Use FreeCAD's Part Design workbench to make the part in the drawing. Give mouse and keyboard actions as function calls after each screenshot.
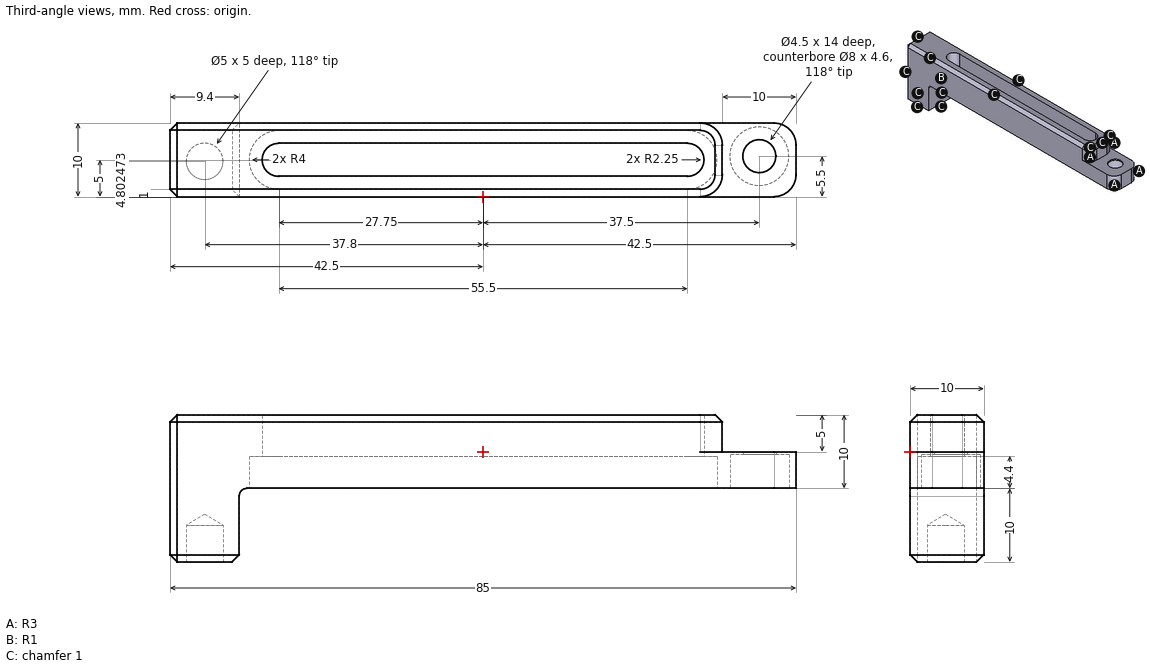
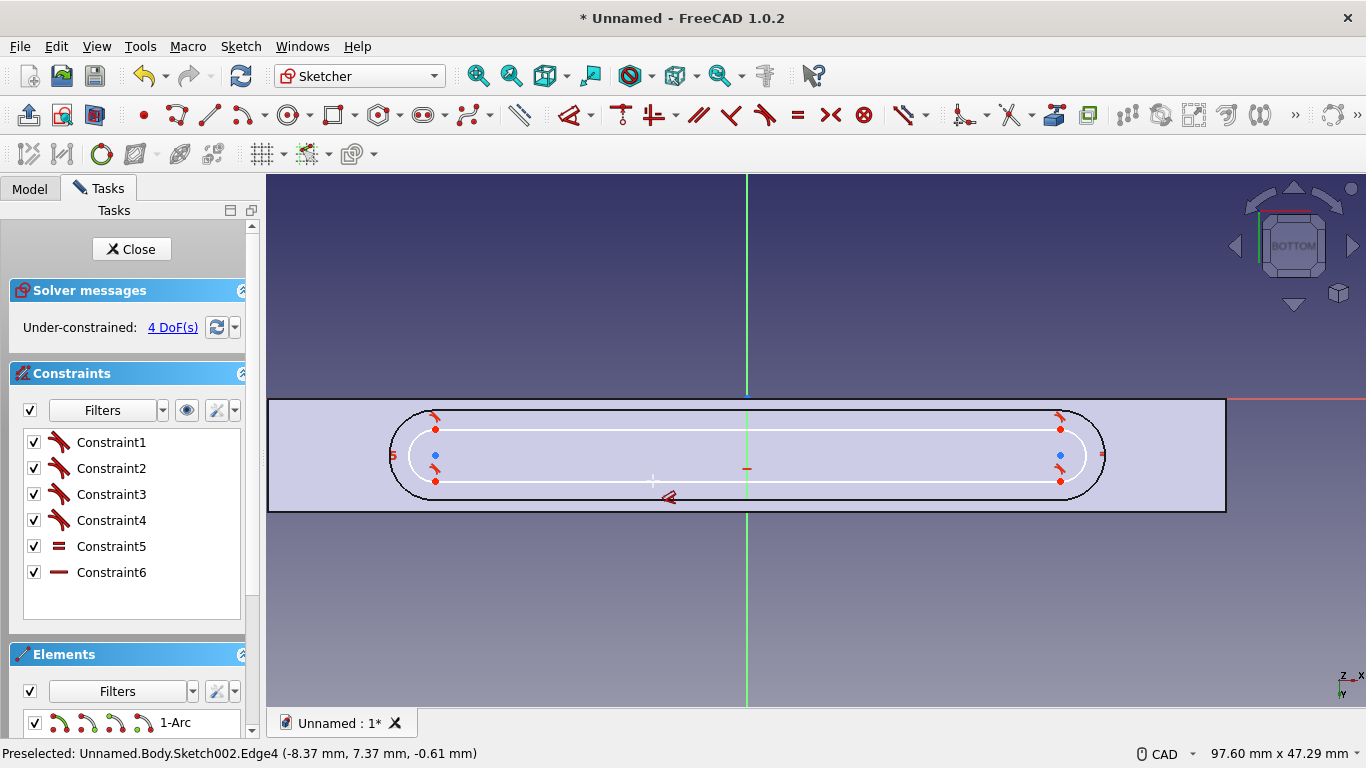
scroll(414, 441, up, 3)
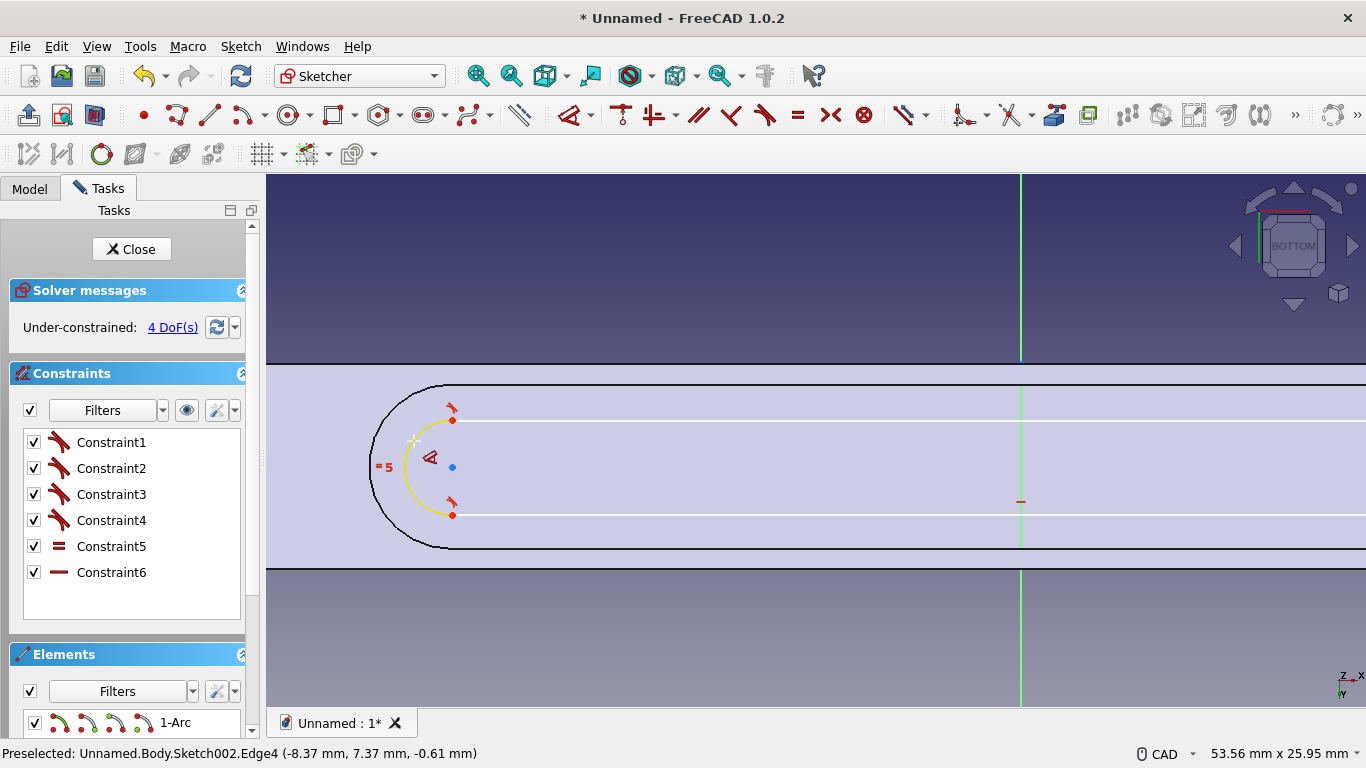
click(414, 440)
click(388, 421)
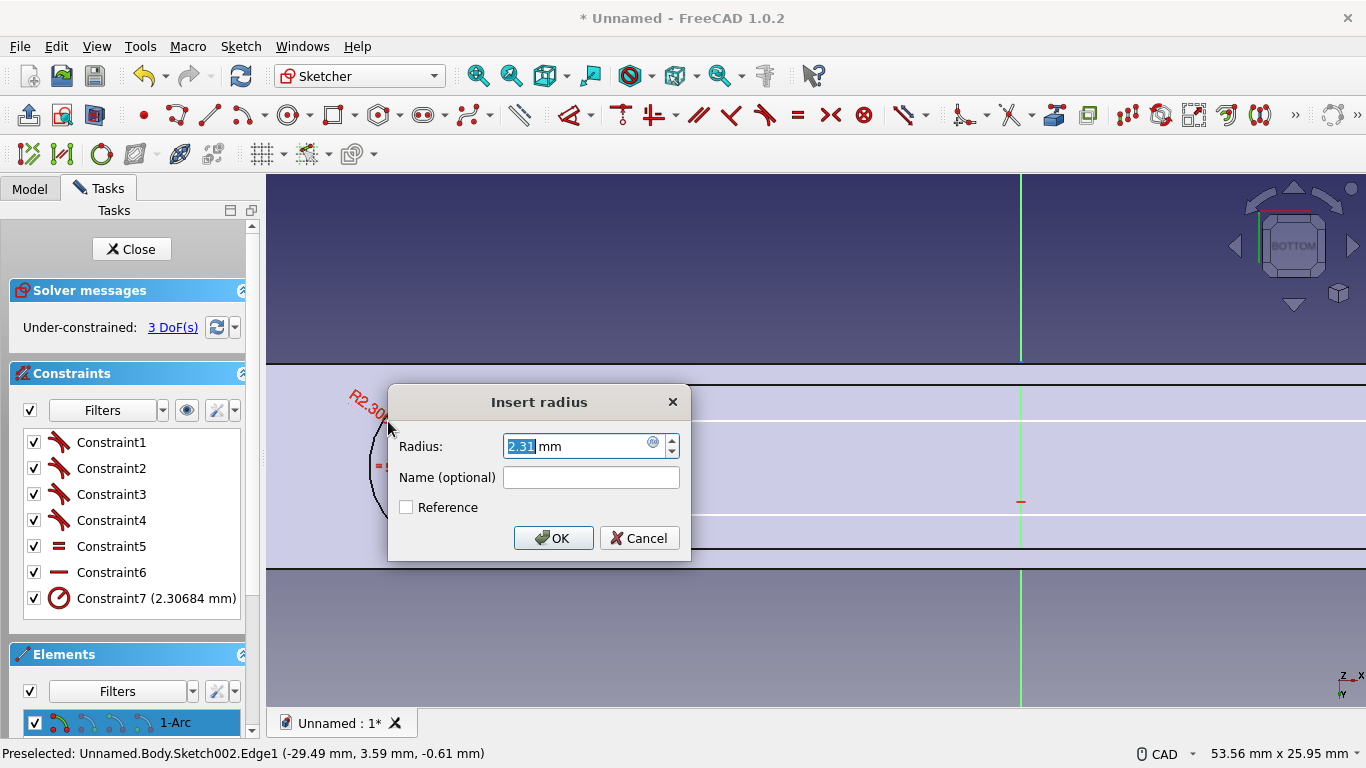
text(2.25)
key(Return)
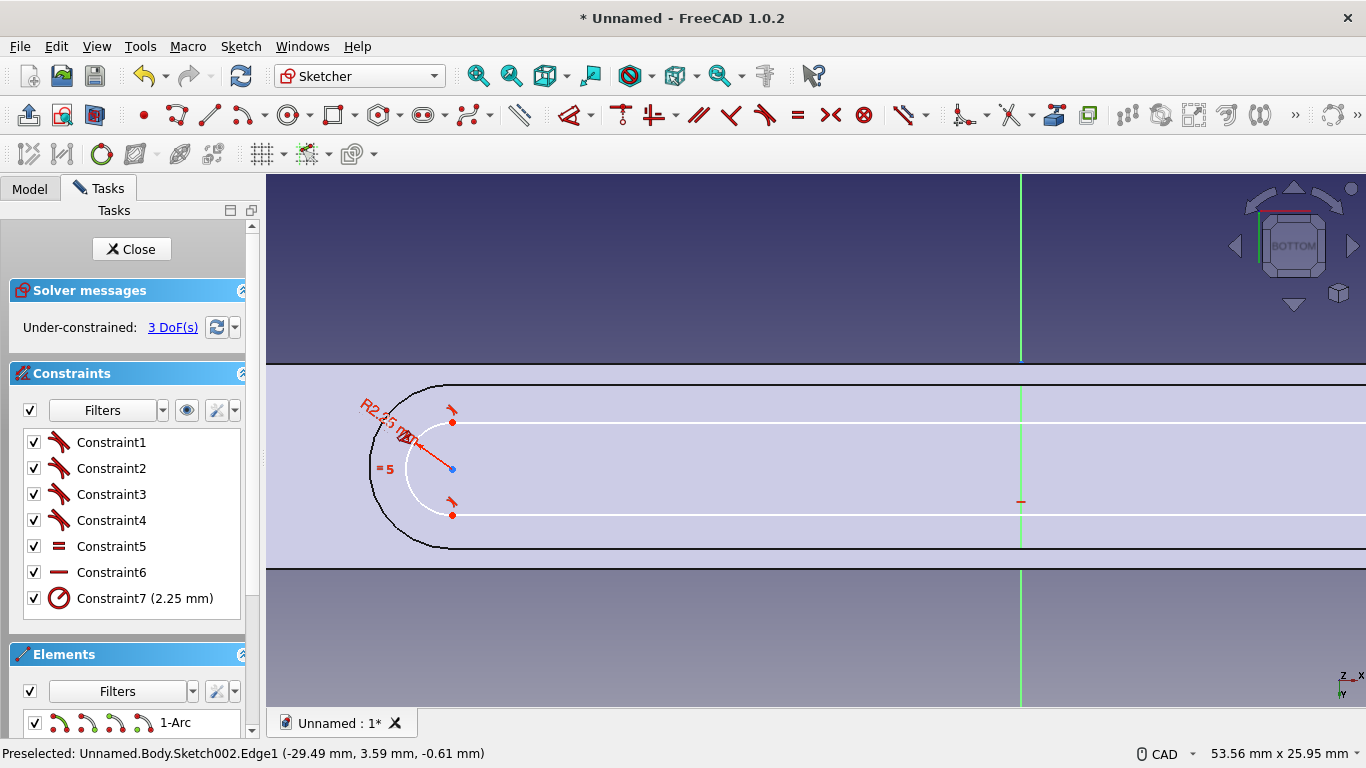
click(452, 469)
click(418, 392)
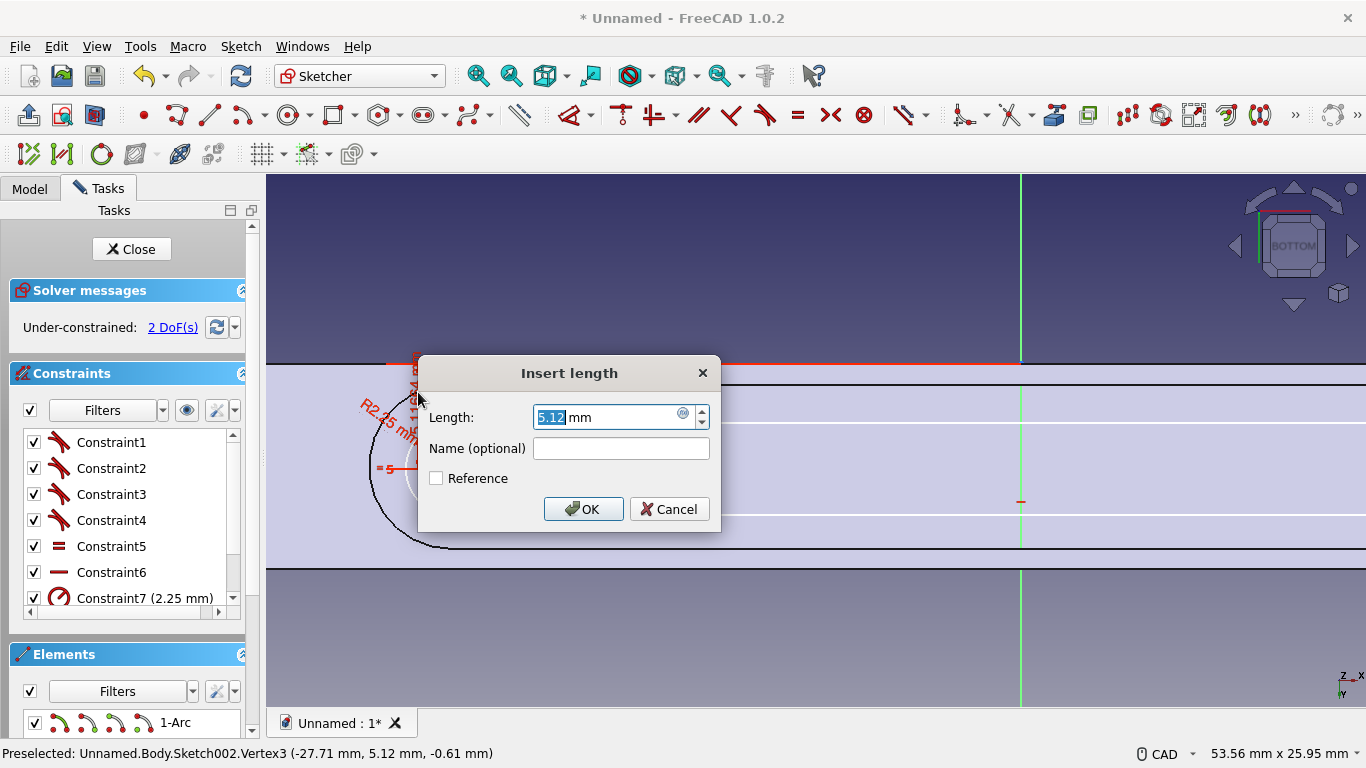
text(5)
key(Return)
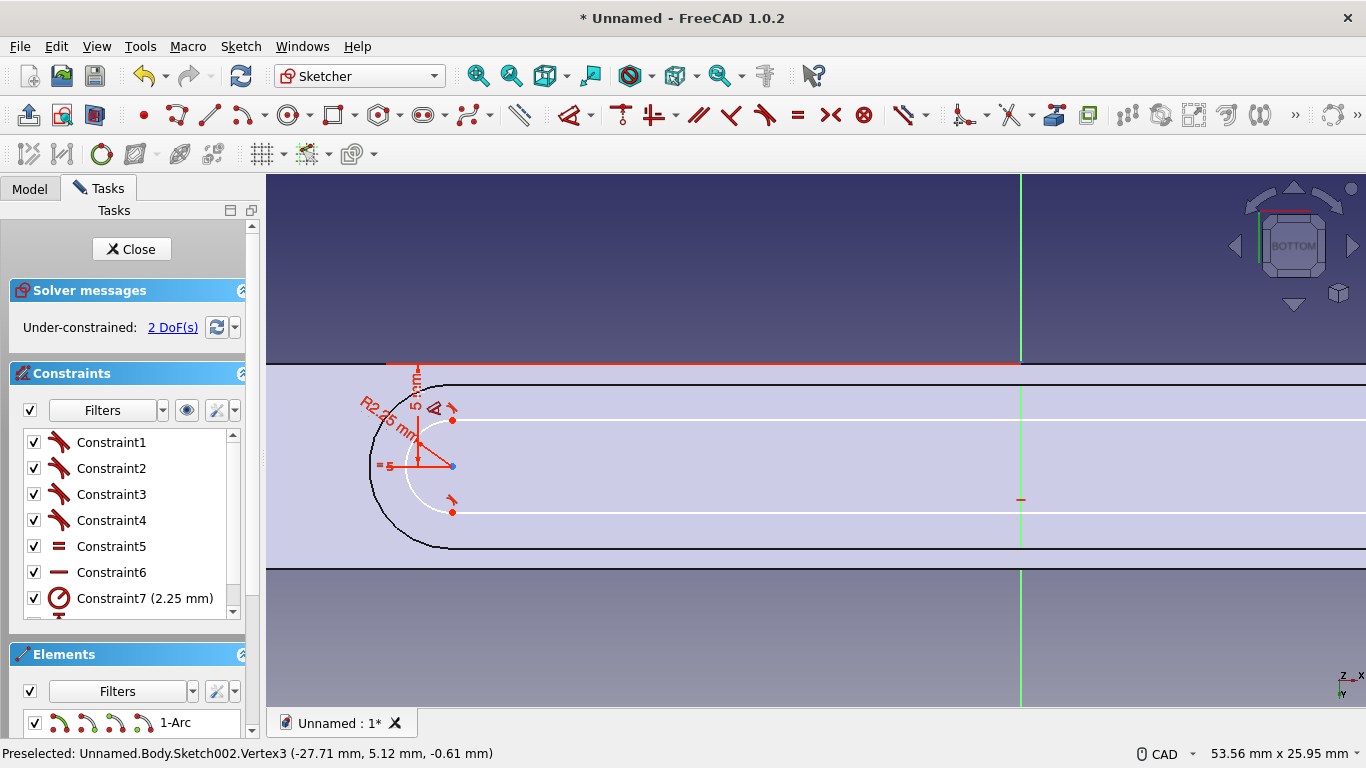
click(794, 420)
click(827, 386)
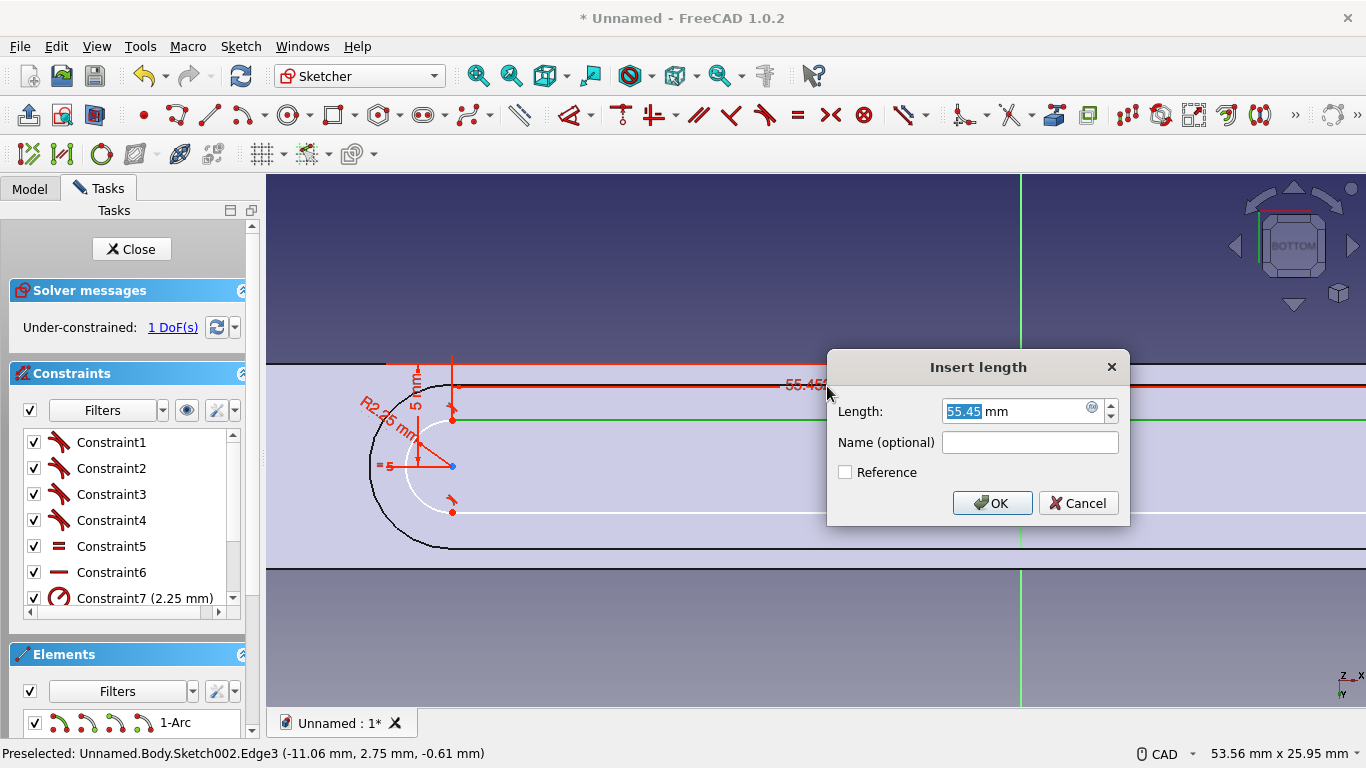
text(55.5)
key(Return)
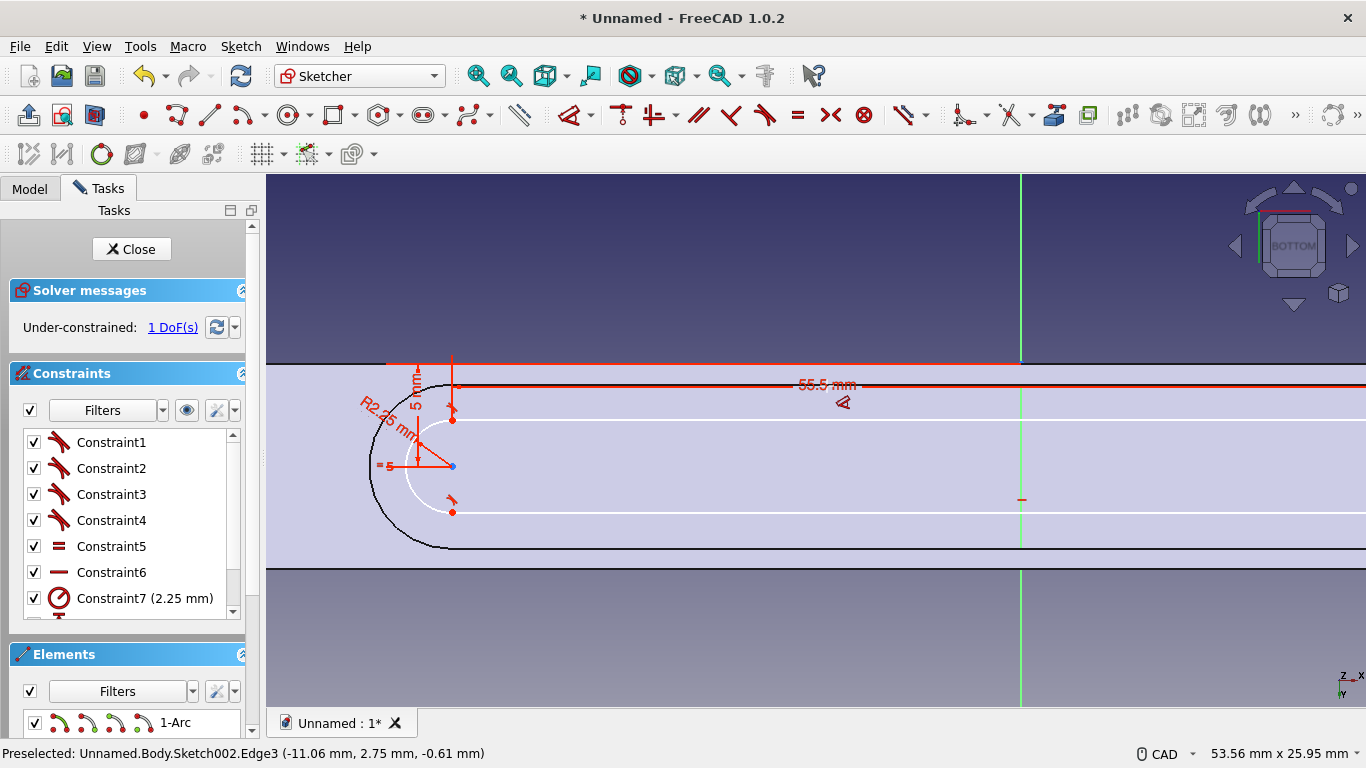
click(452, 420)
click(737, 330)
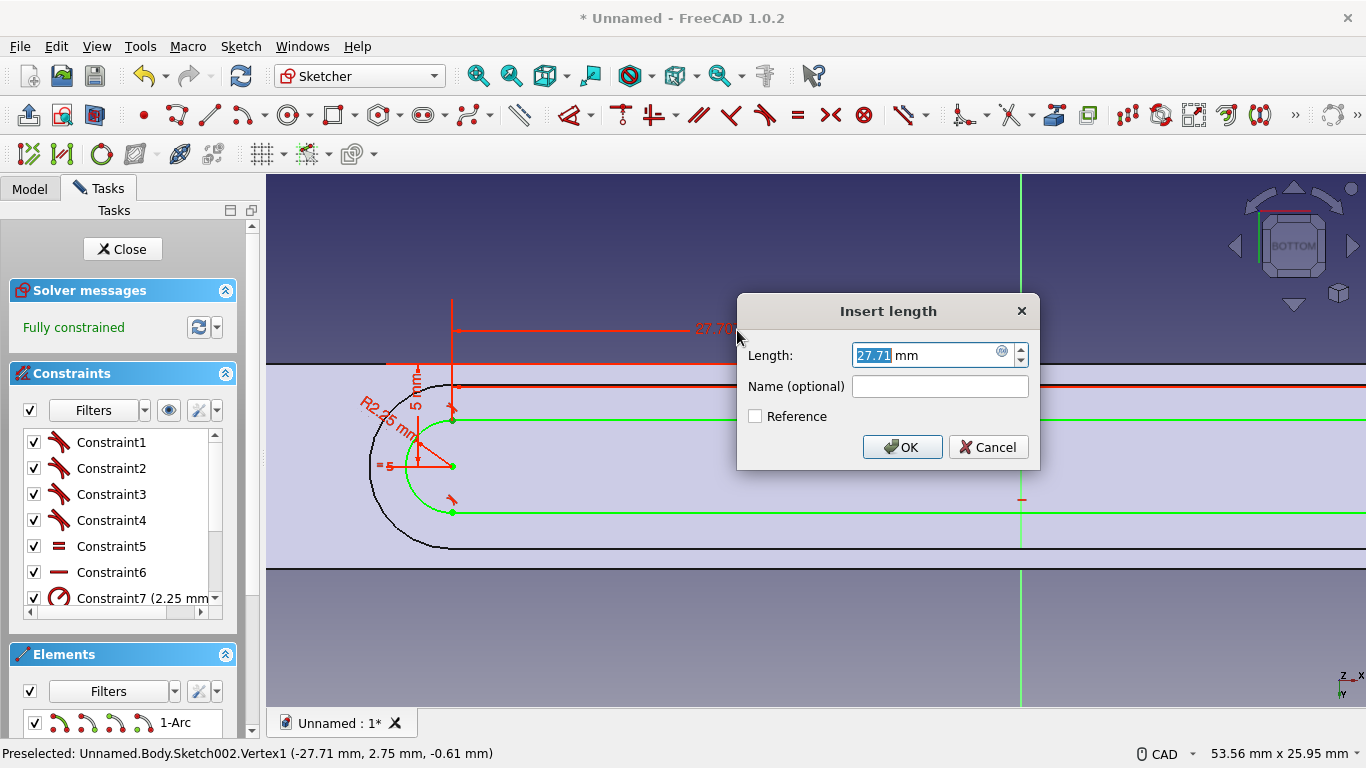
text(27.75)
key(Return)
key(Escape)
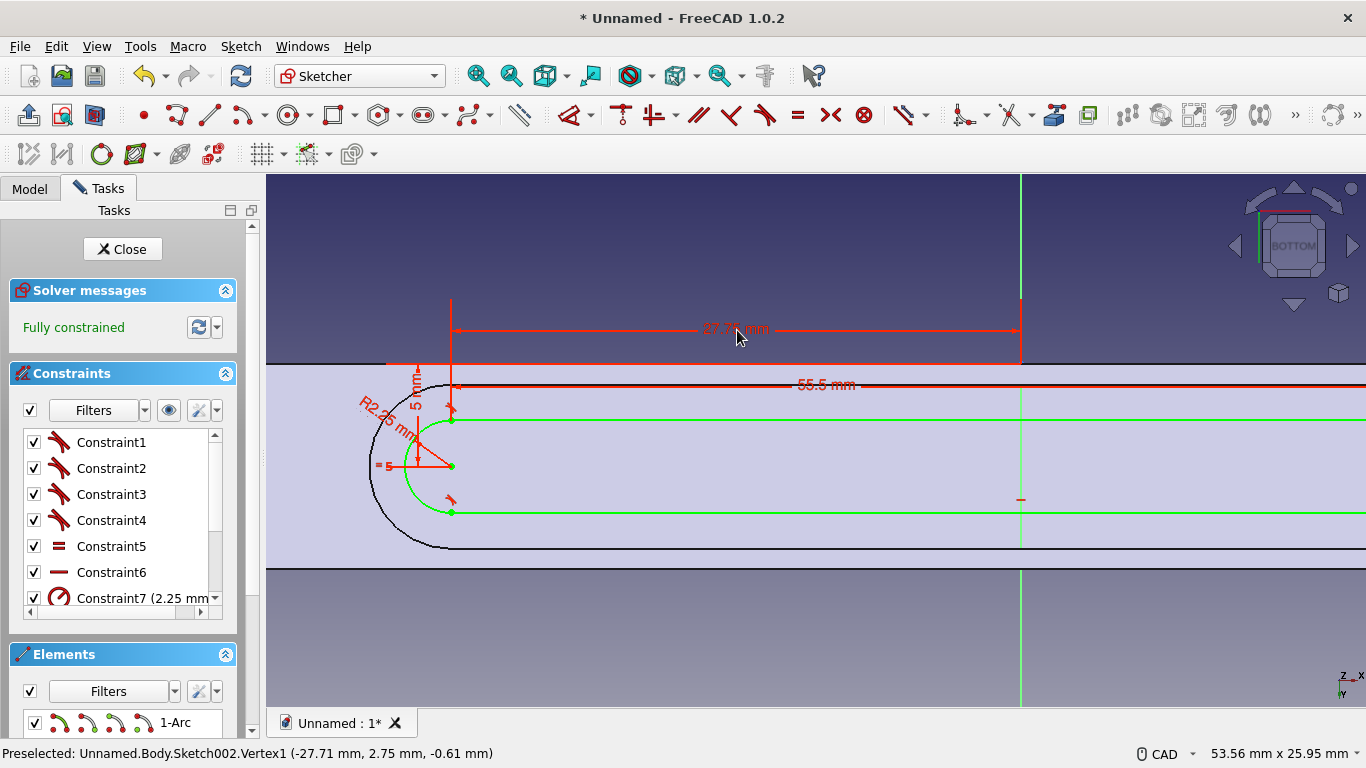
click(123, 249)